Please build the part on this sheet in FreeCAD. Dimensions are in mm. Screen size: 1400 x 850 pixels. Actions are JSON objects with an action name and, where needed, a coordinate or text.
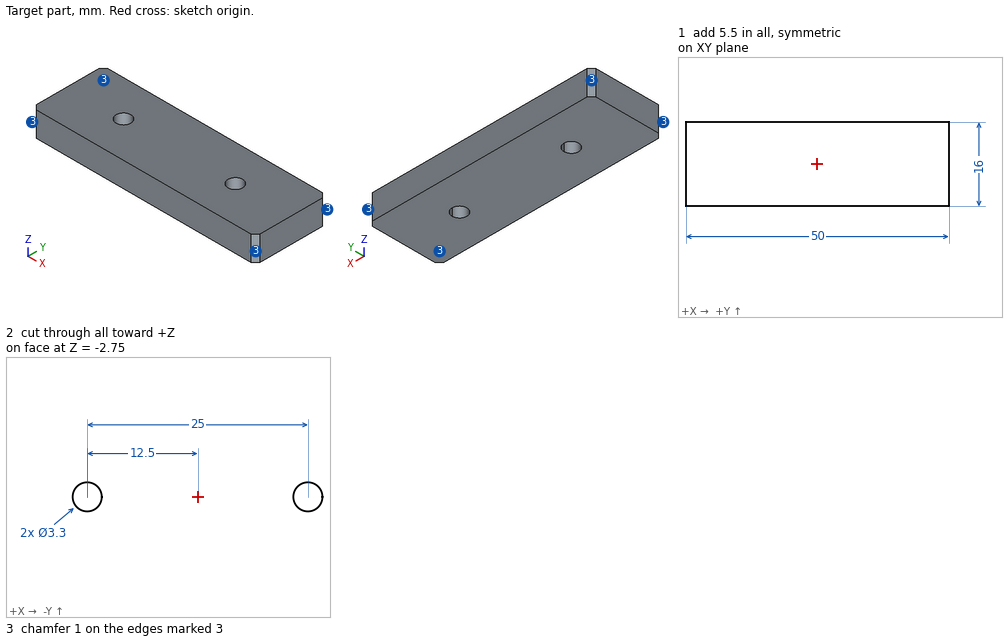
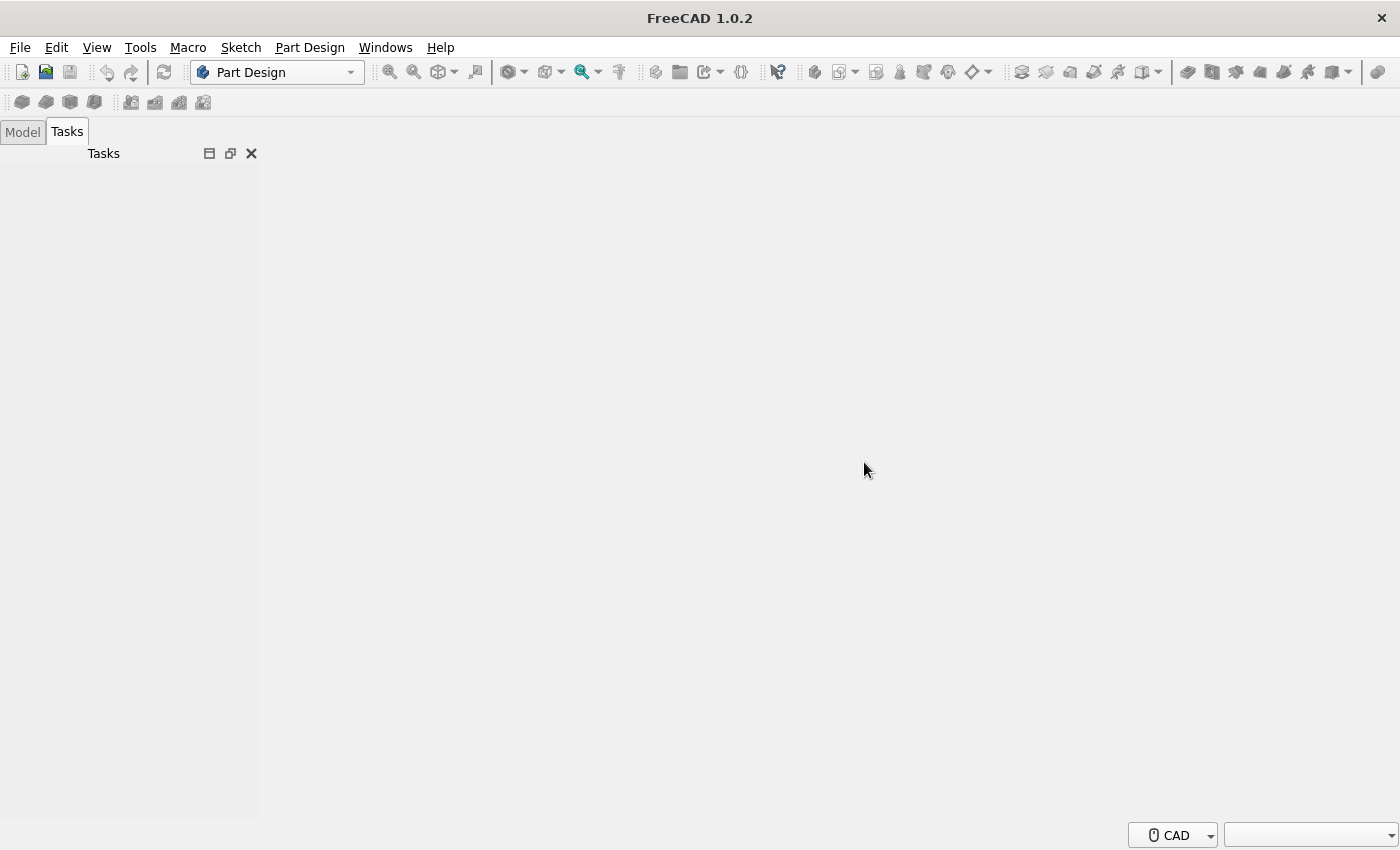
{"action": "left_click", "coordinate": [22, 72]}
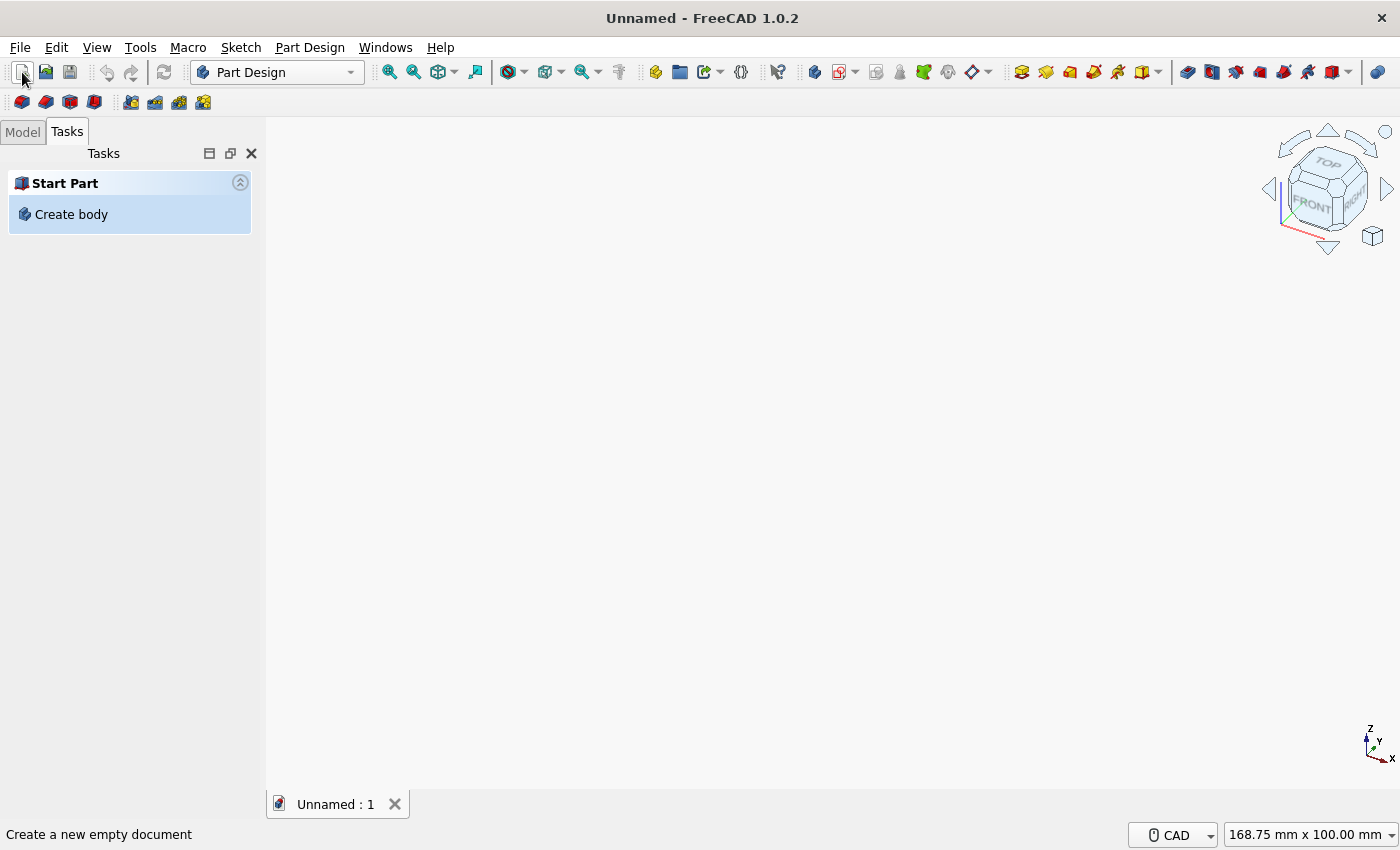
{"action": "left_click", "coordinate": [840, 72]}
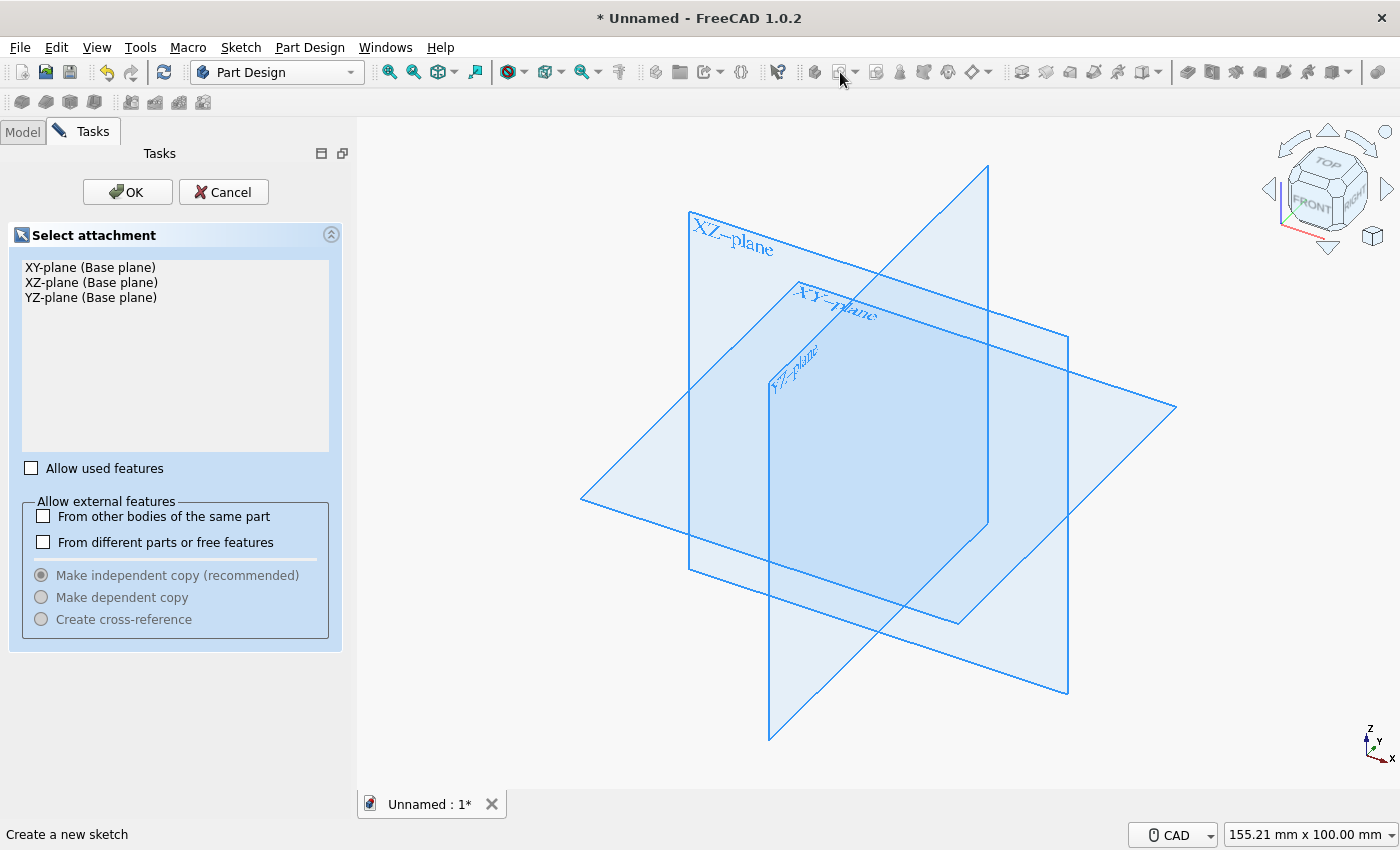
{"action": "left_click", "coordinate": [82, 268]}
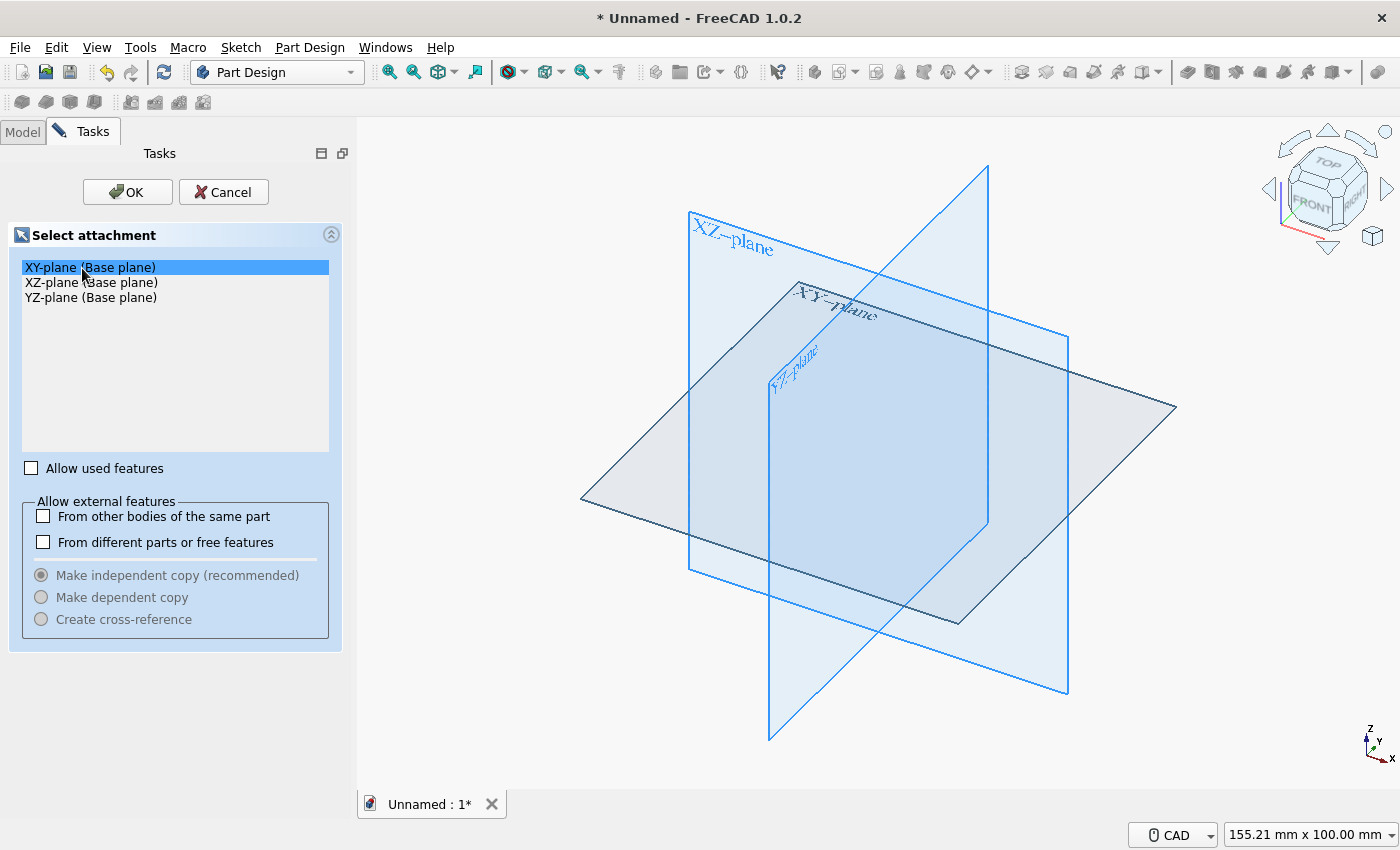
{"action": "left_click", "coordinate": [128, 192]}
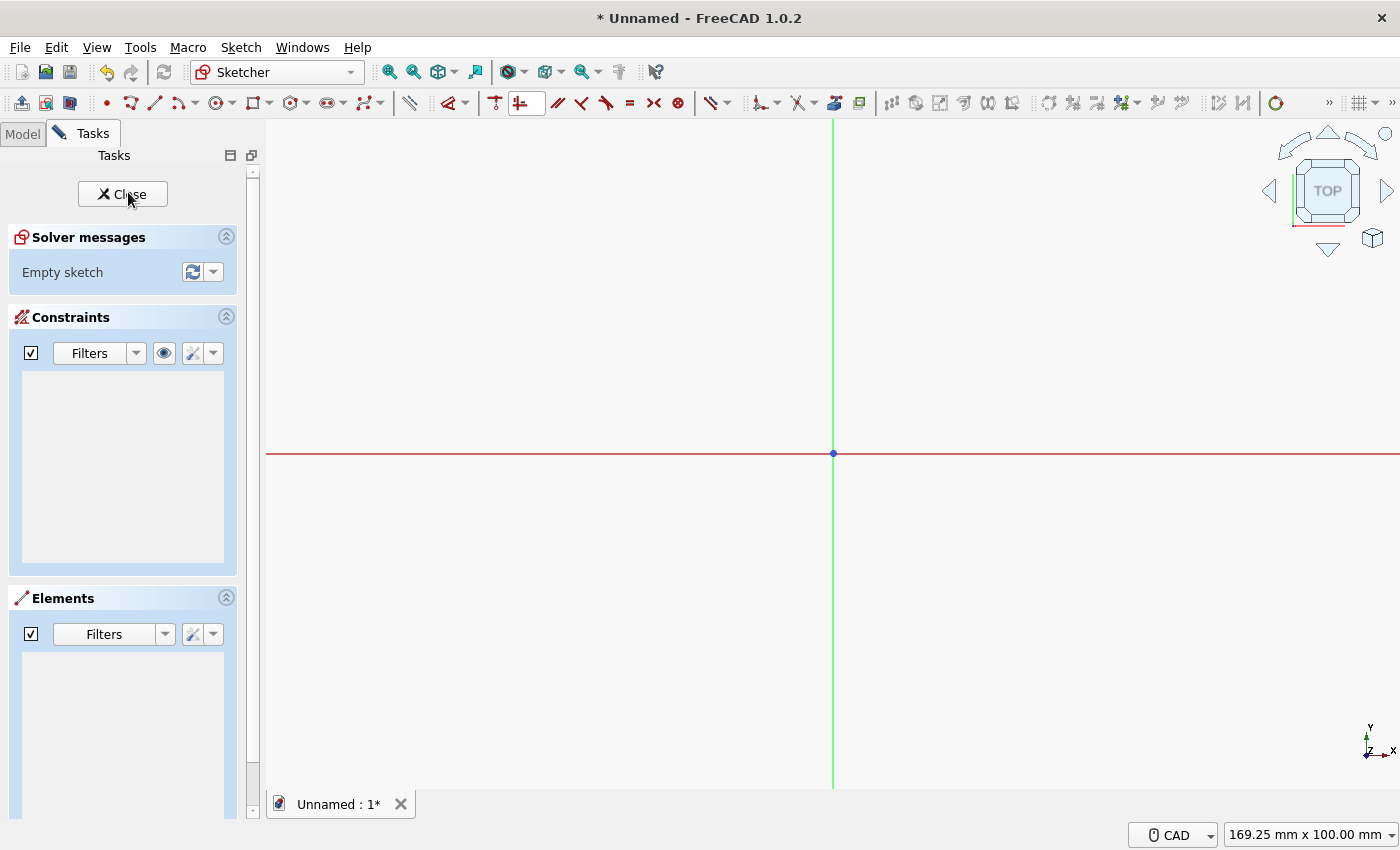
{"action": "scroll", "coordinate": [916, 454], "scroll_direction": "up", "scroll_amount": 3}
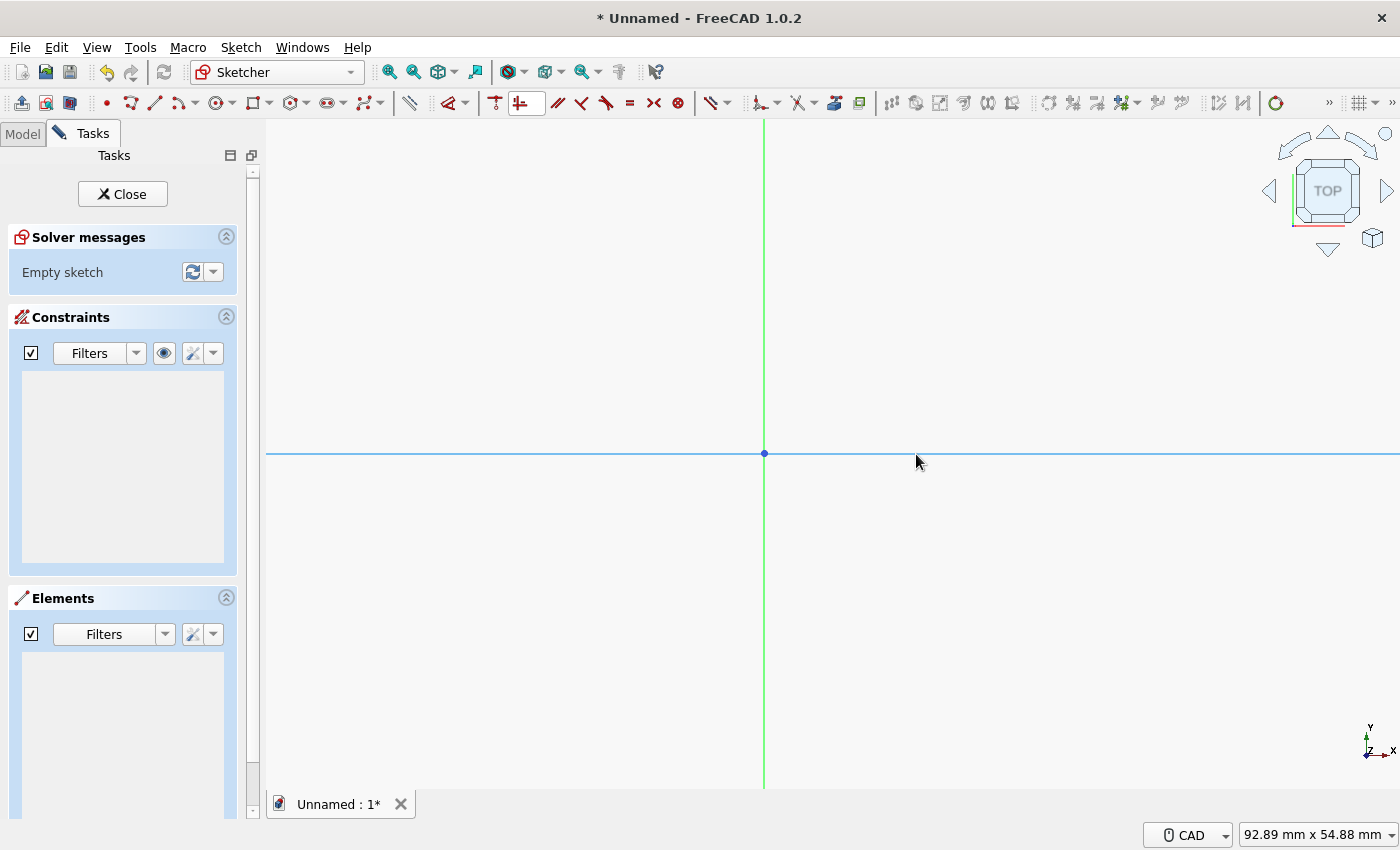
{"action": "key", "text": "g v"}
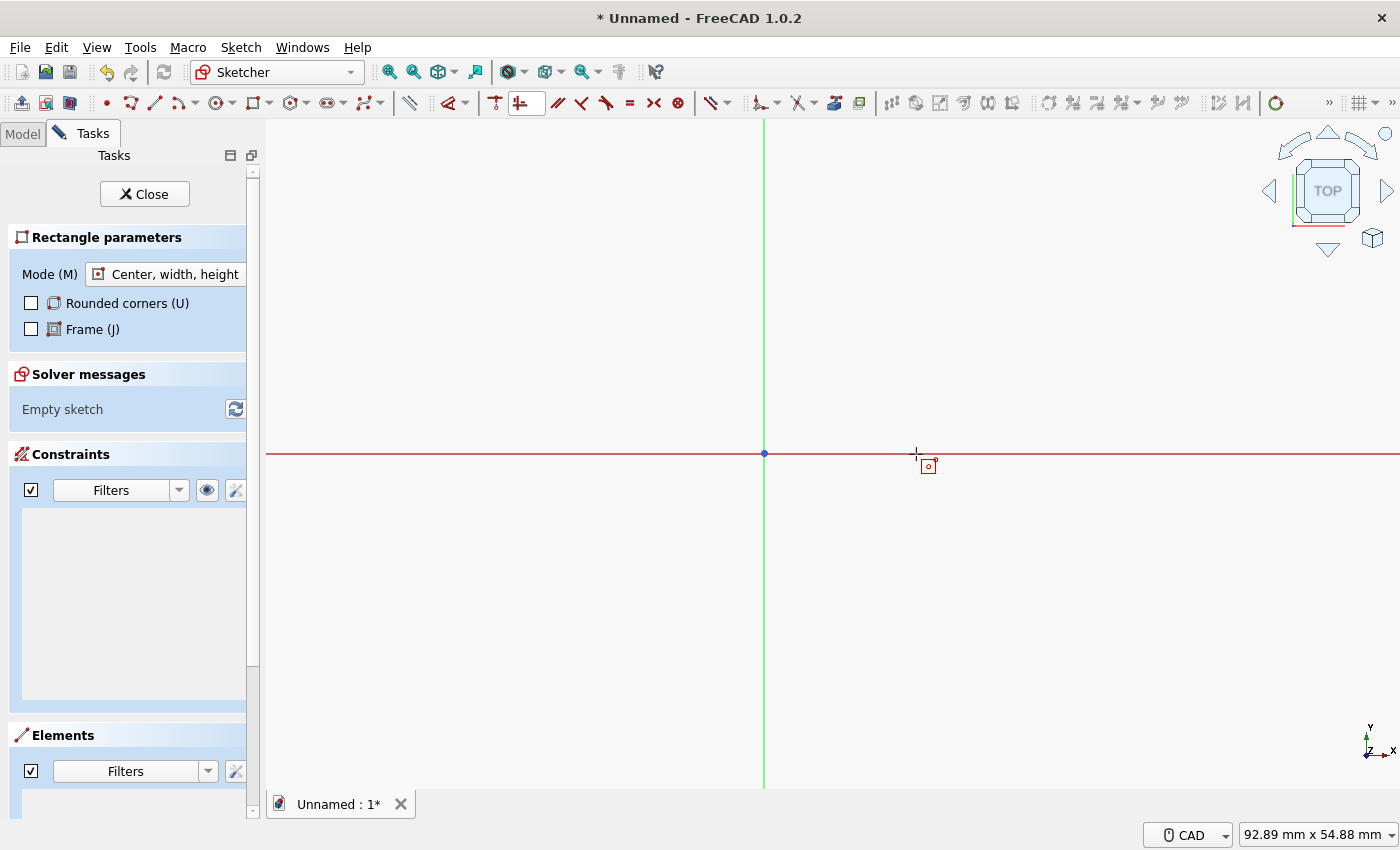
{"action": "left_click", "coordinate": [764, 454]}
{"action": "left_click", "coordinate": [1069, 356]}
{"action": "key", "text": "Escape"}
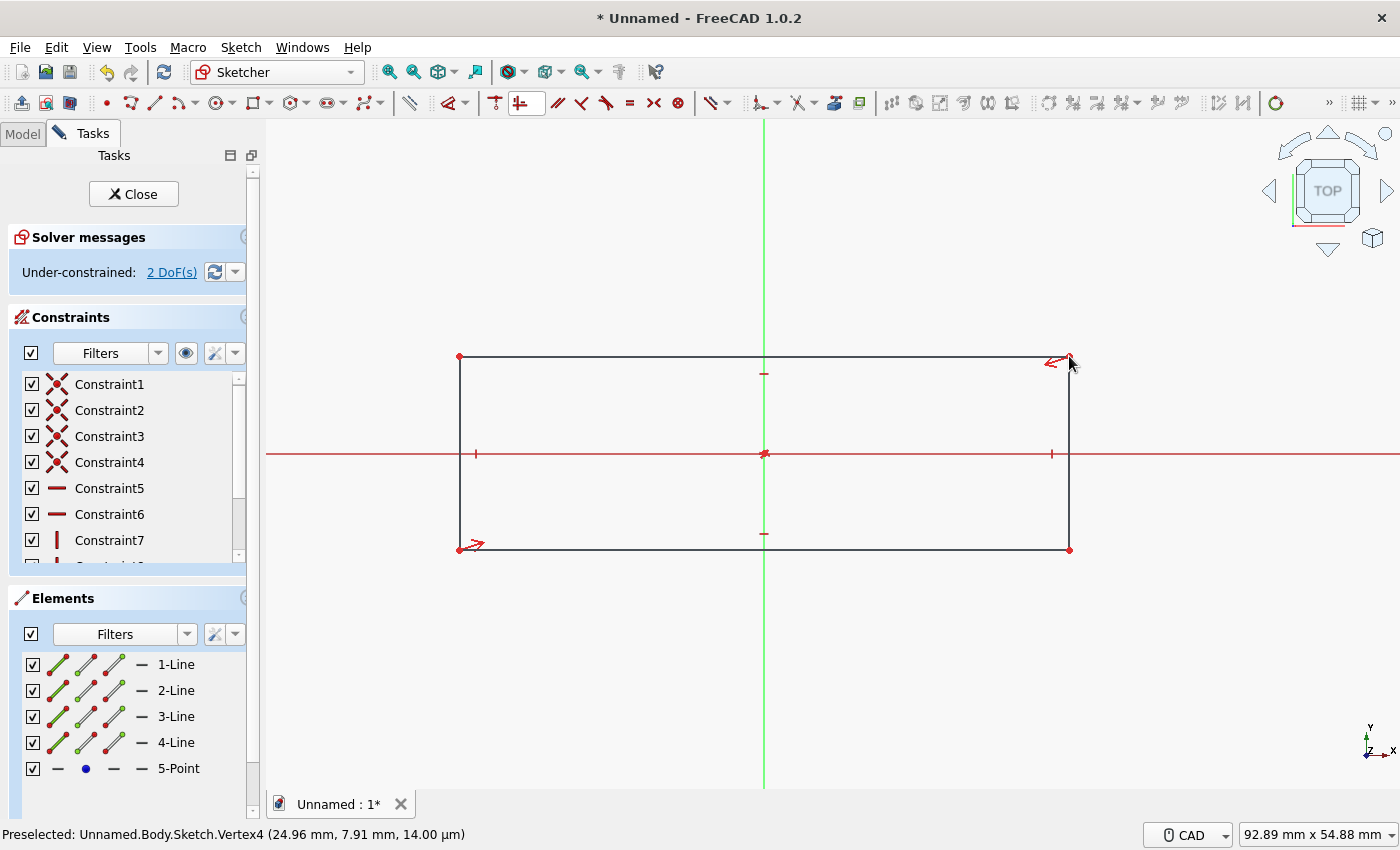
{"action": "left_click", "coordinate": [448, 104]}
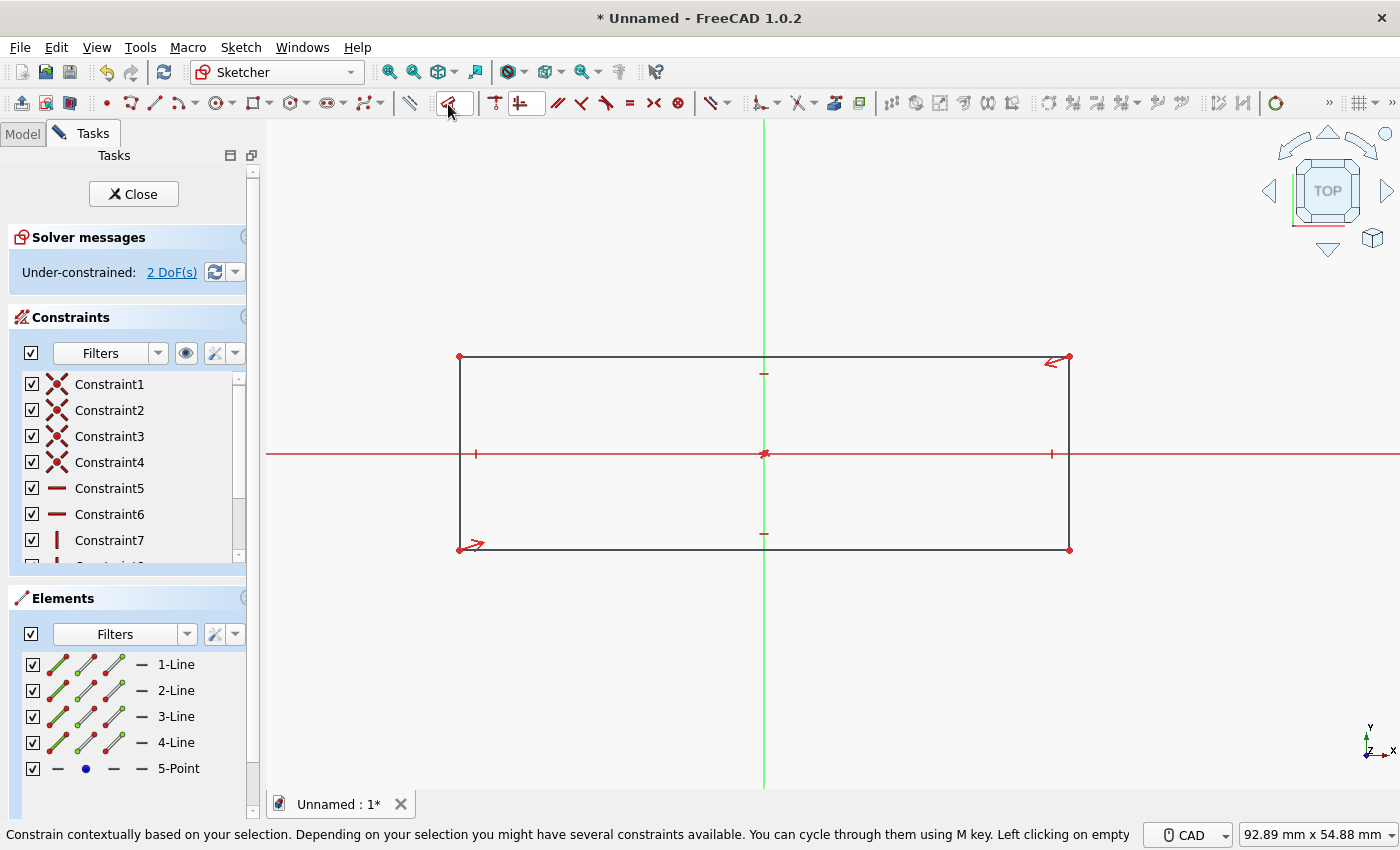
{"action": "left_click", "coordinate": [642, 550]}
{"action": "left_click", "coordinate": [624, 584]}